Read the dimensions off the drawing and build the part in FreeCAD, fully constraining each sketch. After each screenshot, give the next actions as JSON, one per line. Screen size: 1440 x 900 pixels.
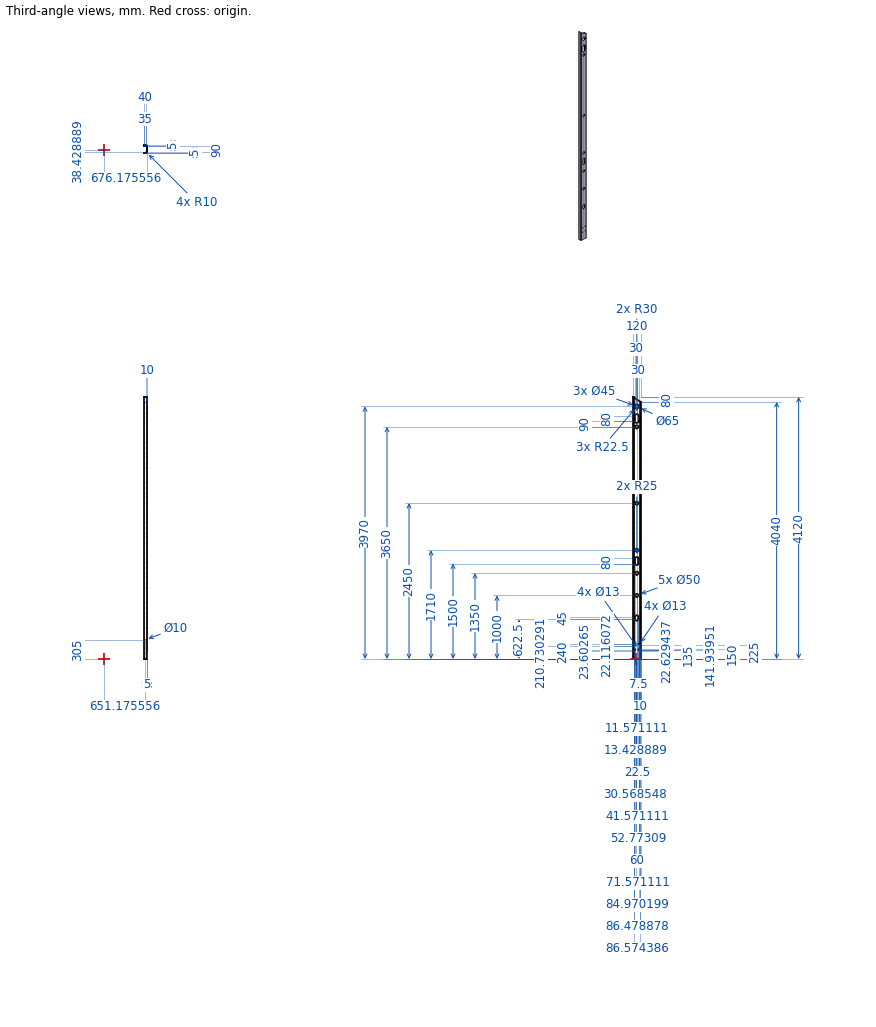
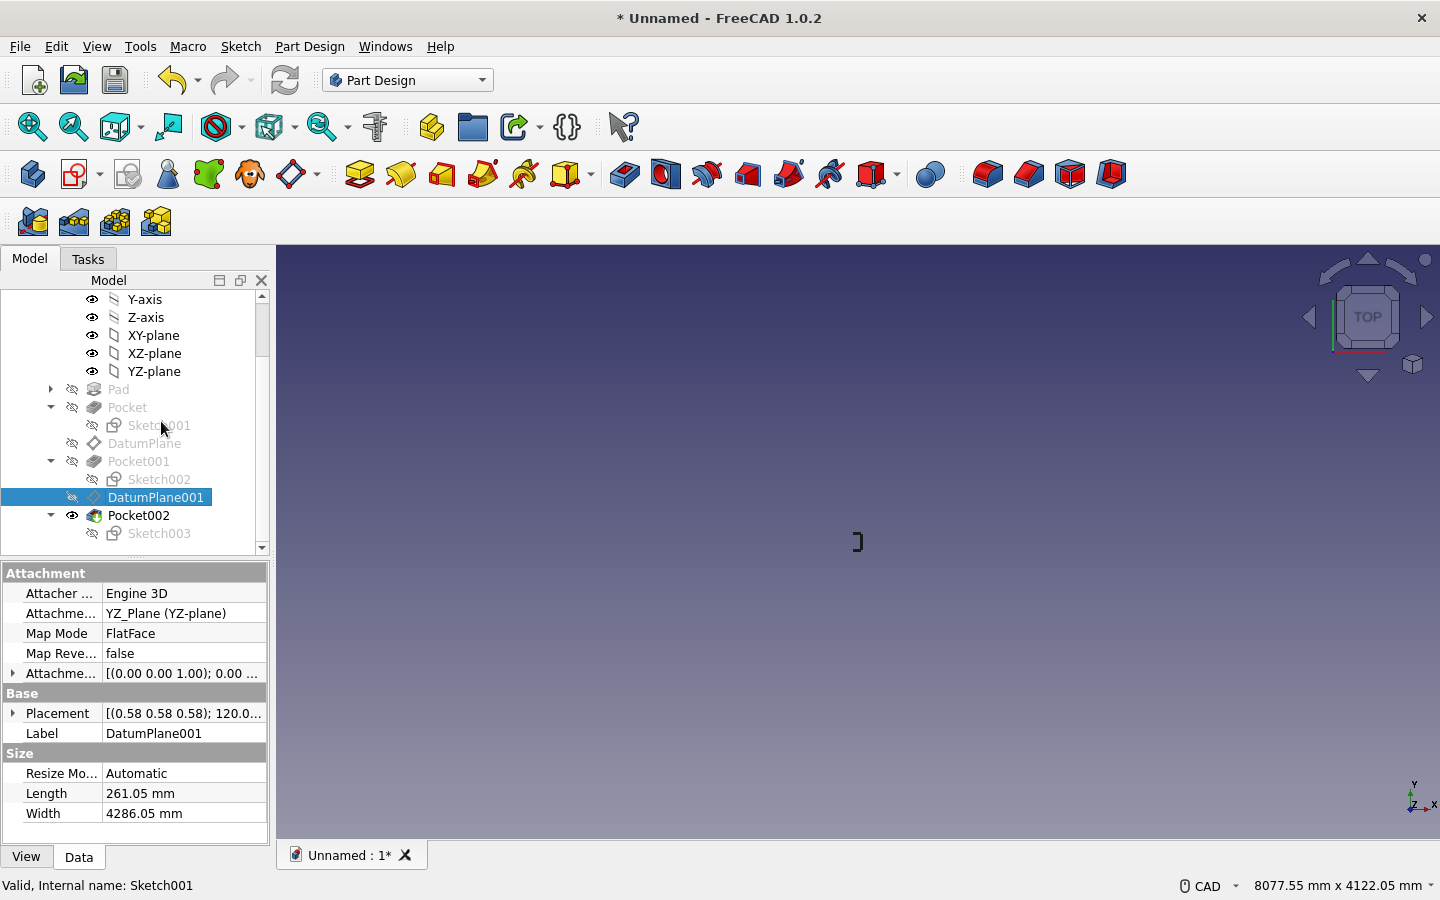
{"action": "scroll", "coordinate": [161, 421], "scroll_direction": "up", "scroll_amount": 15}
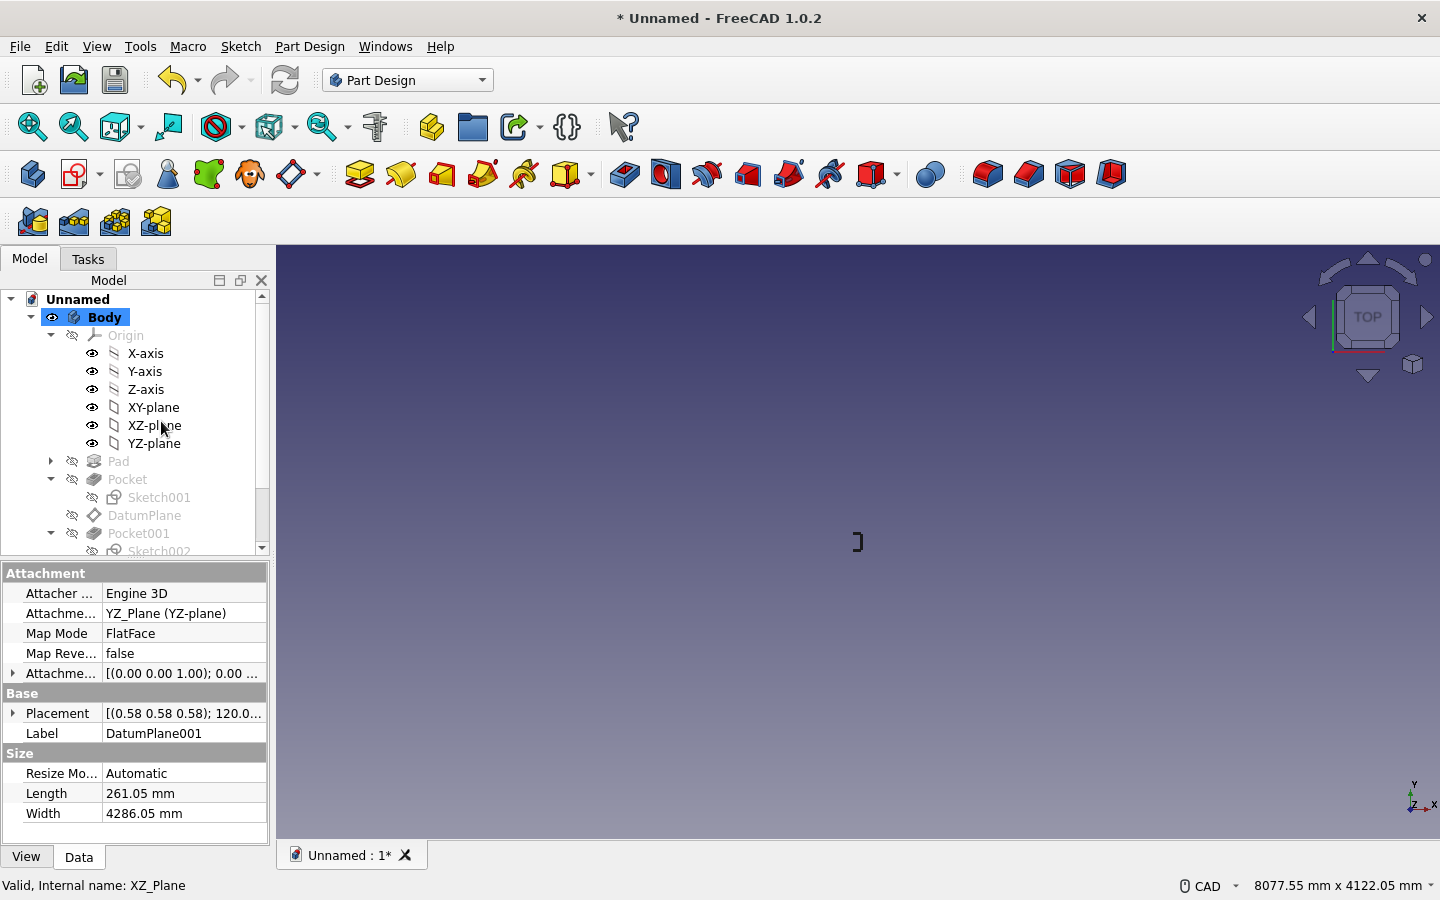
{"action": "left_click", "coordinate": [137, 443]}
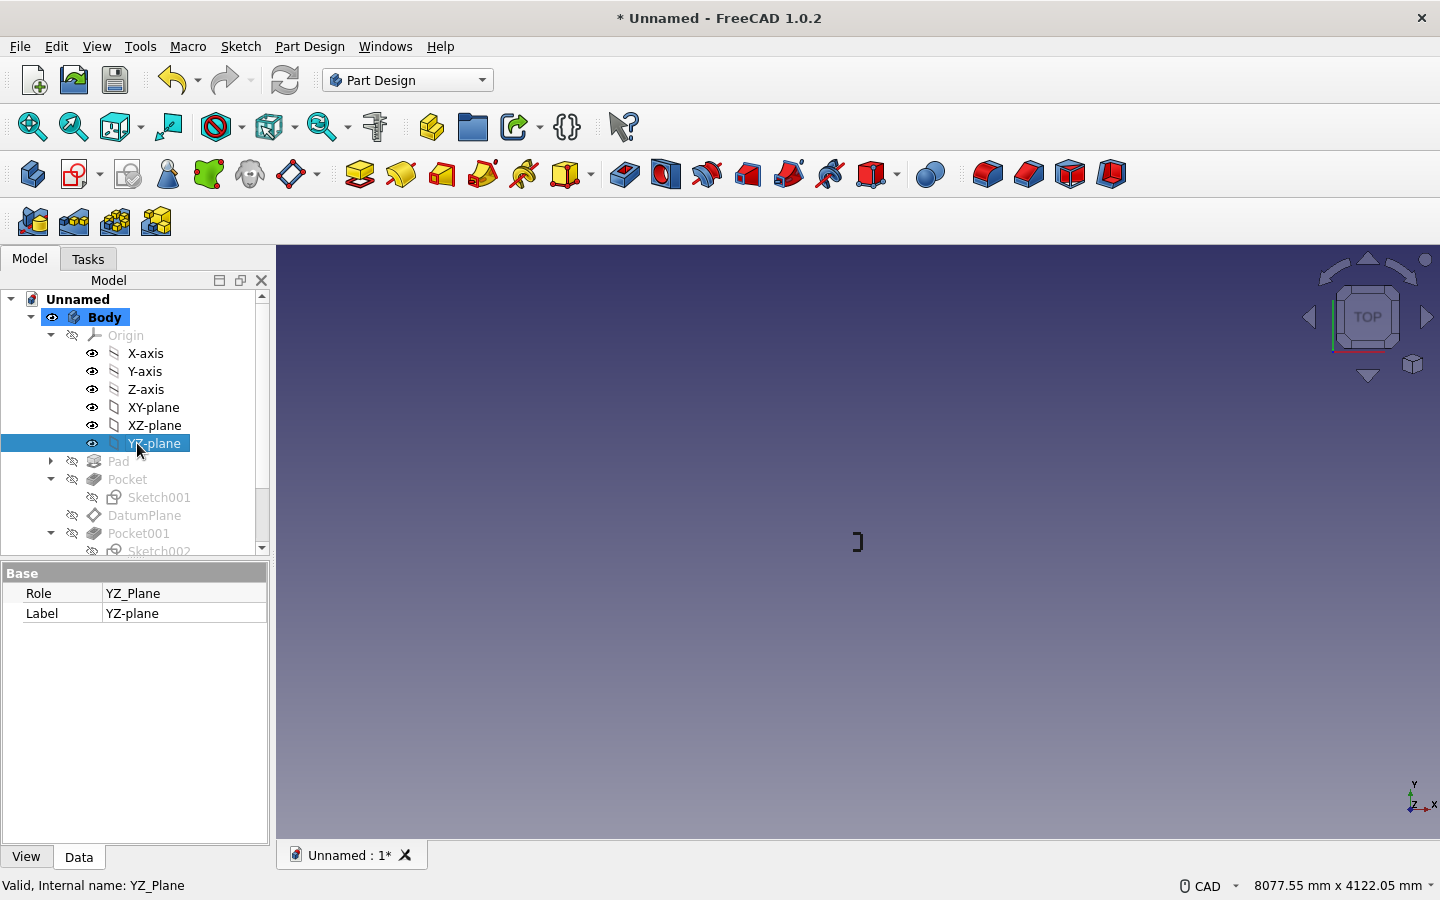
{"action": "left_click", "coordinate": [290, 174]}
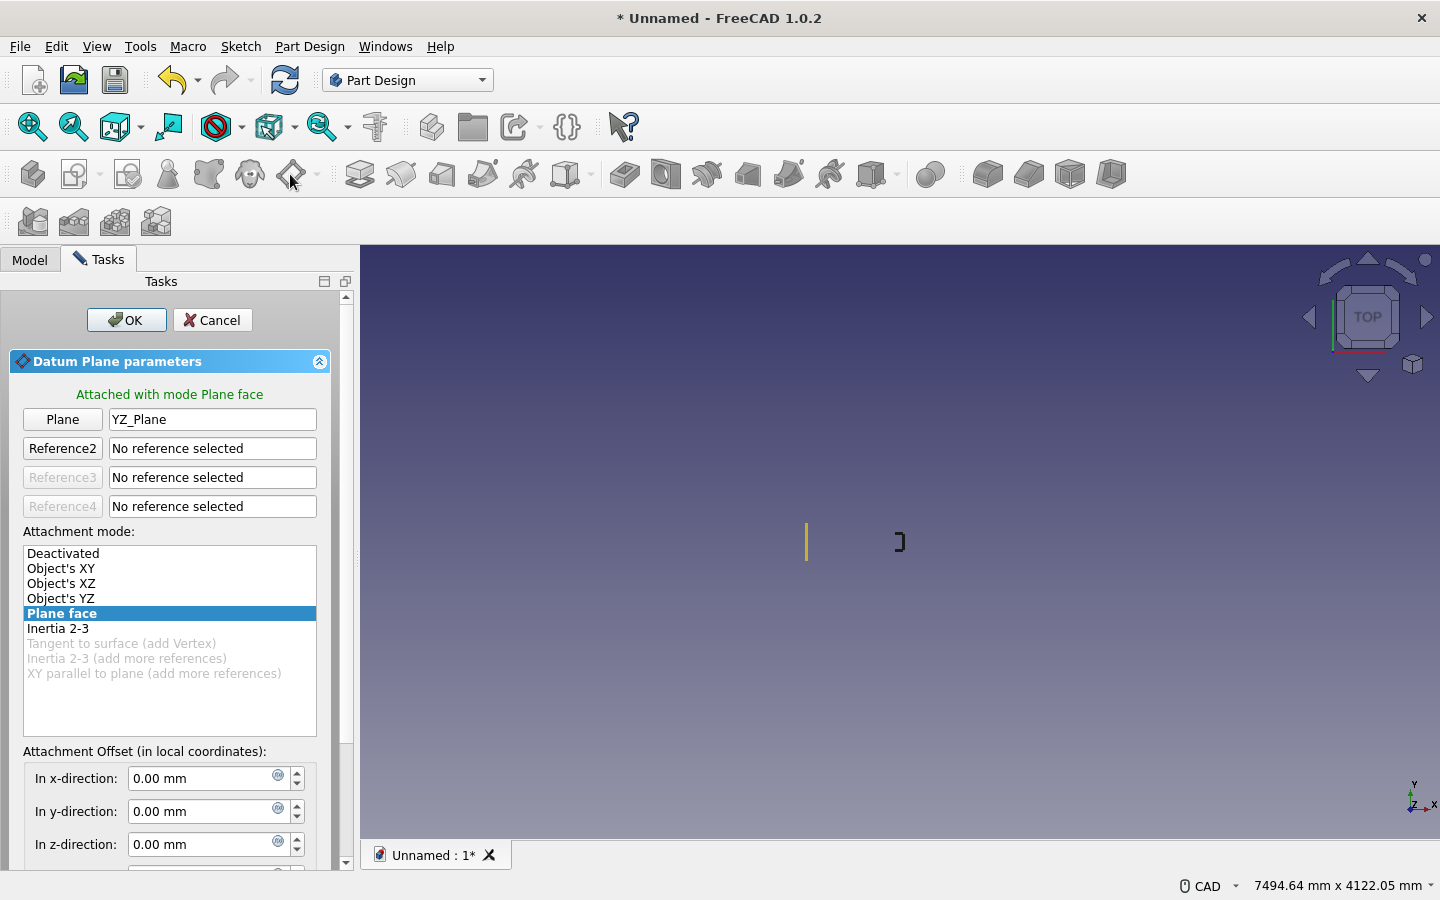
{"action": "triple_click", "coordinate": [210, 844]}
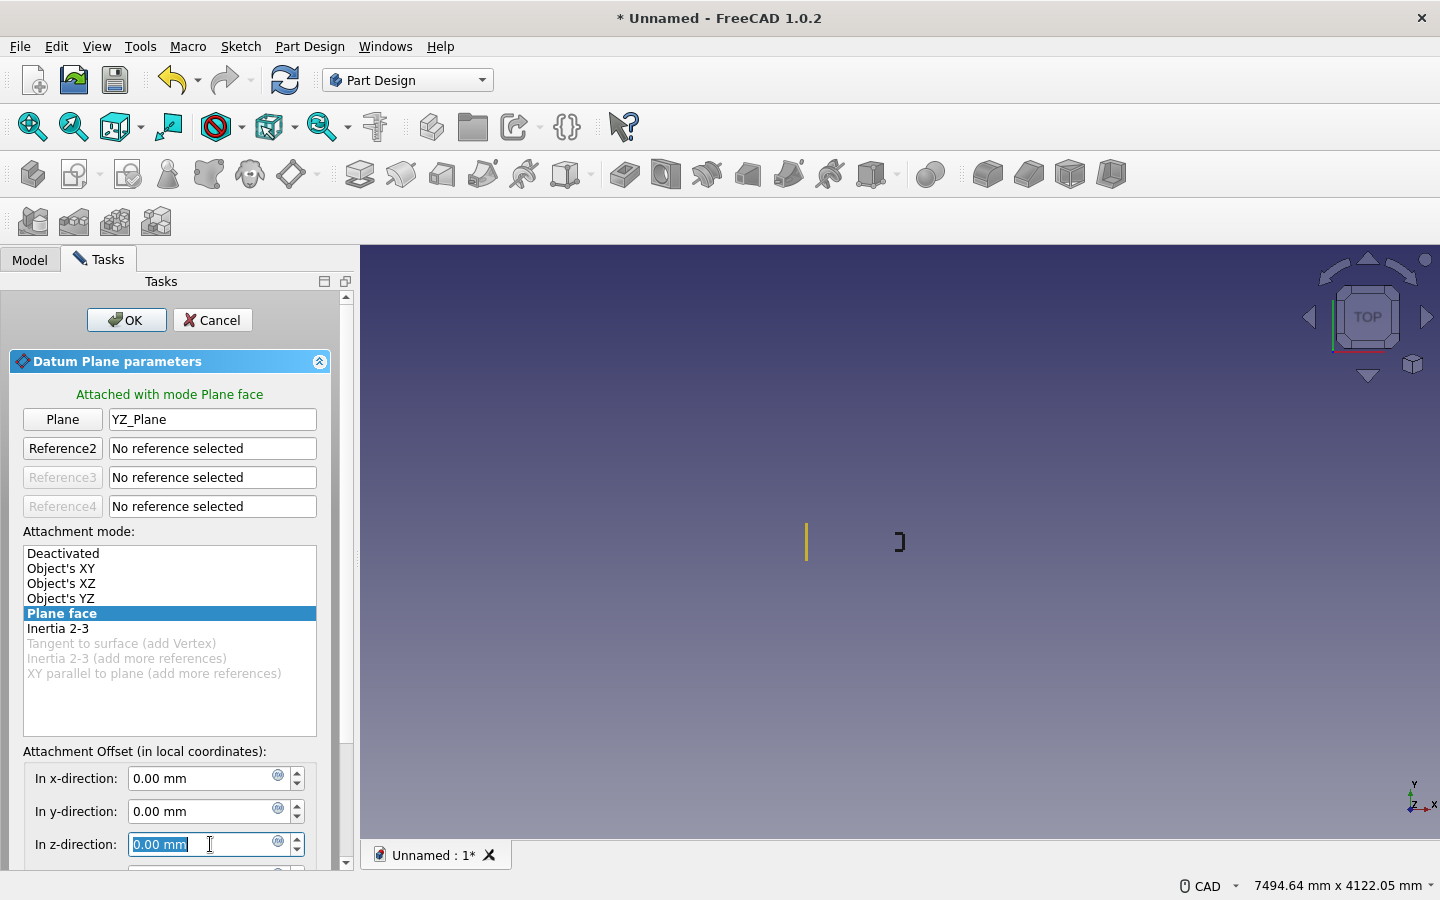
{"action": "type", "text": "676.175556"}
{"action": "key", "text": "Tab"}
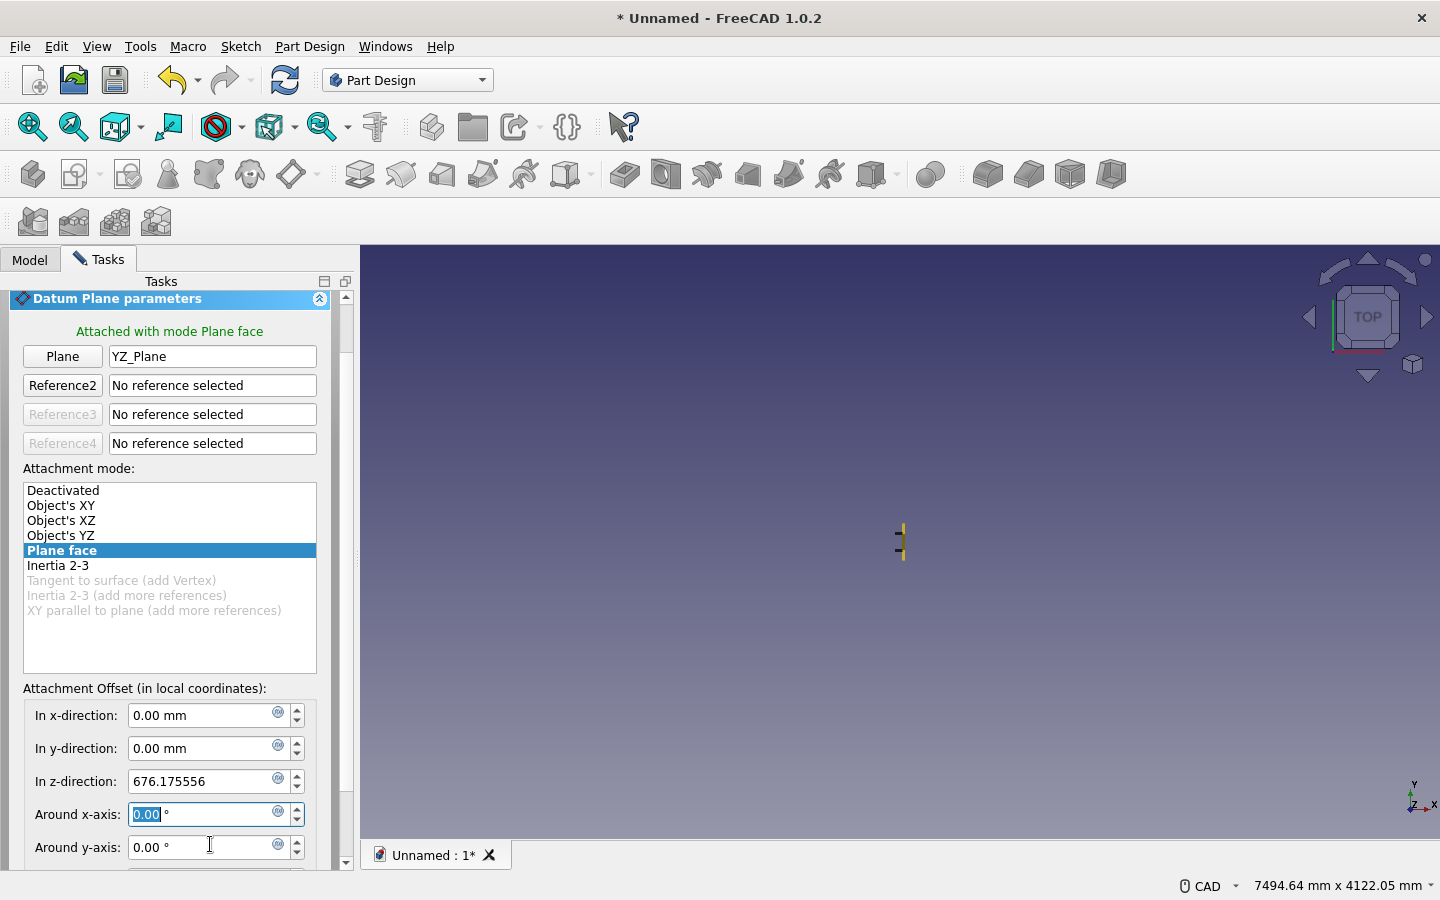
{"action": "scroll", "coordinate": [346, 580], "scroll_direction": "up", "scroll_amount": 2}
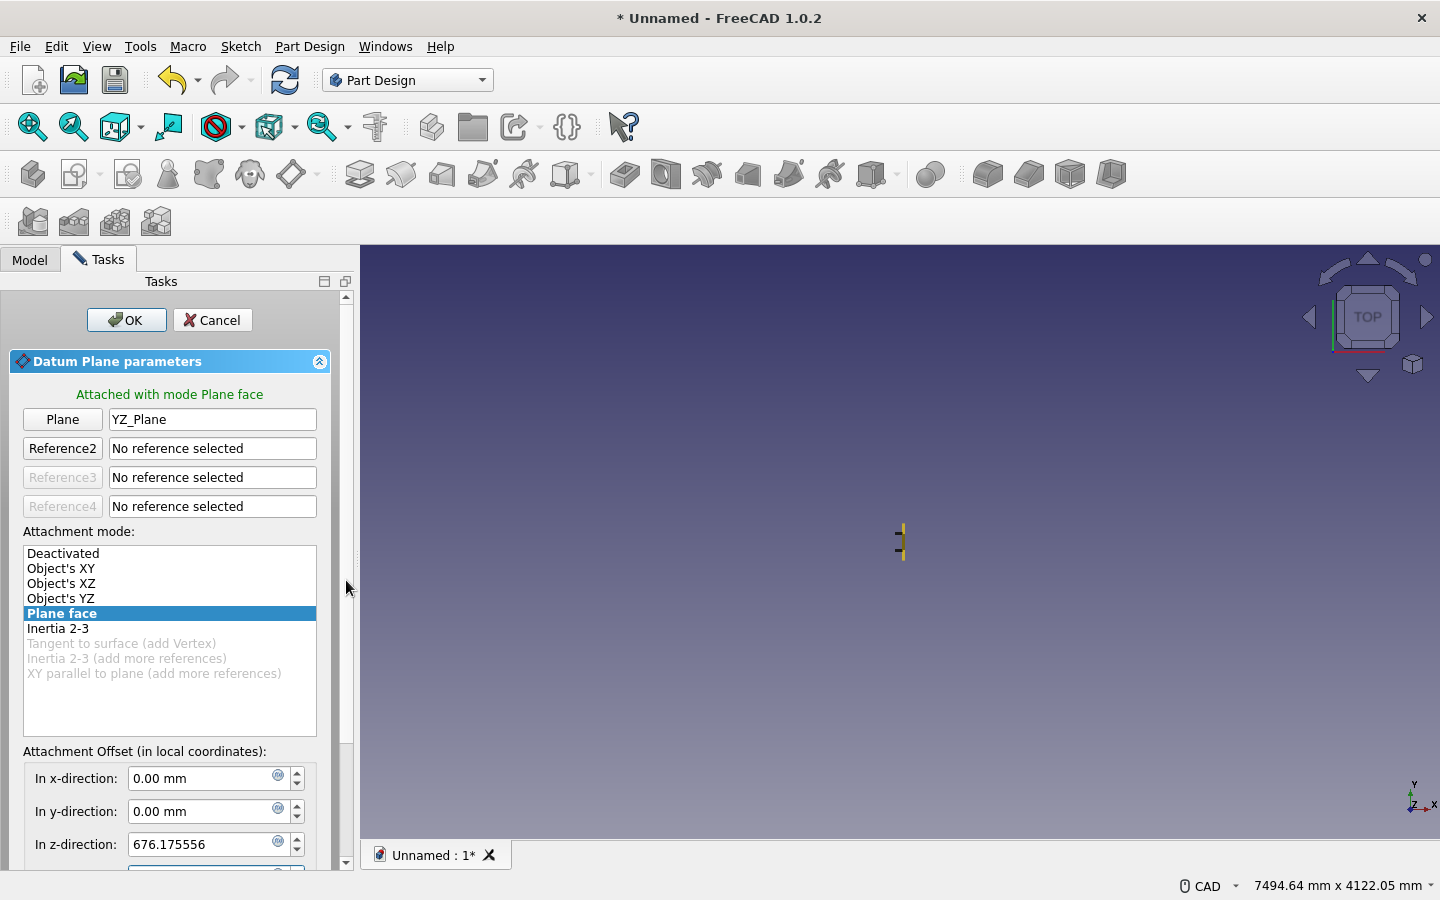
{"action": "left_click", "coordinate": [127, 320]}